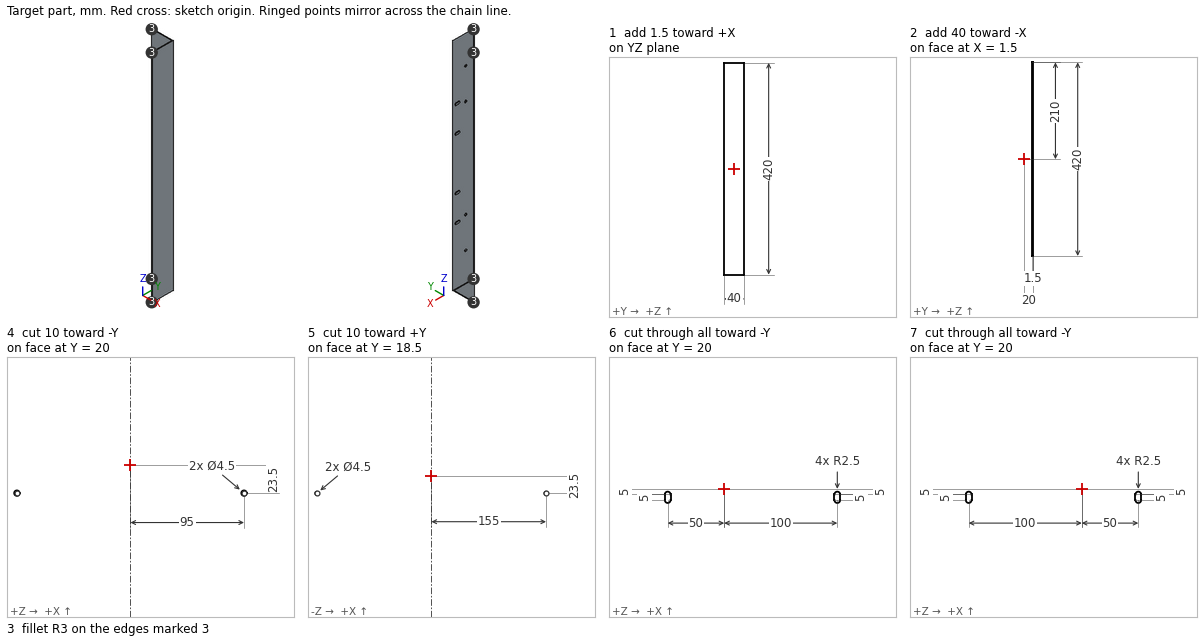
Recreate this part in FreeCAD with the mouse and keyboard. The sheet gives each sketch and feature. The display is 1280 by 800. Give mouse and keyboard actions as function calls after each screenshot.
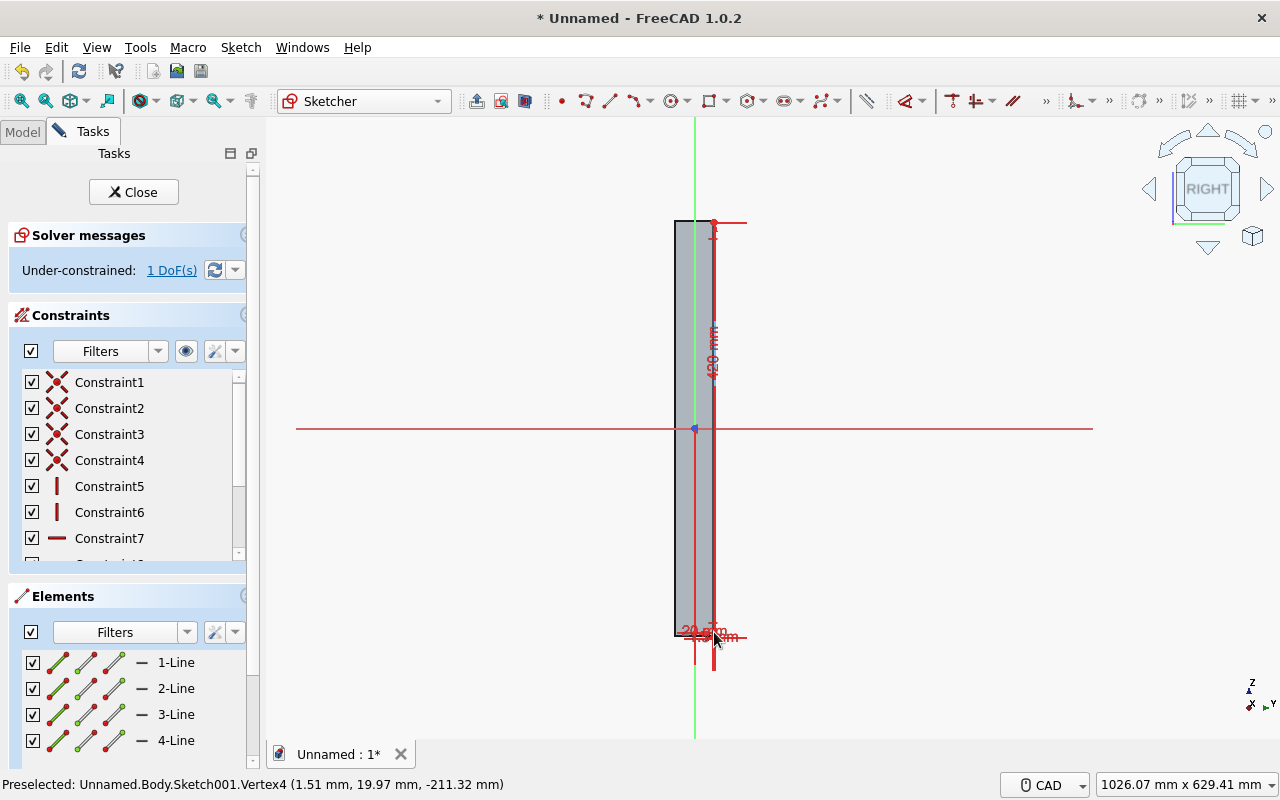
scroll(713, 223, up, 11)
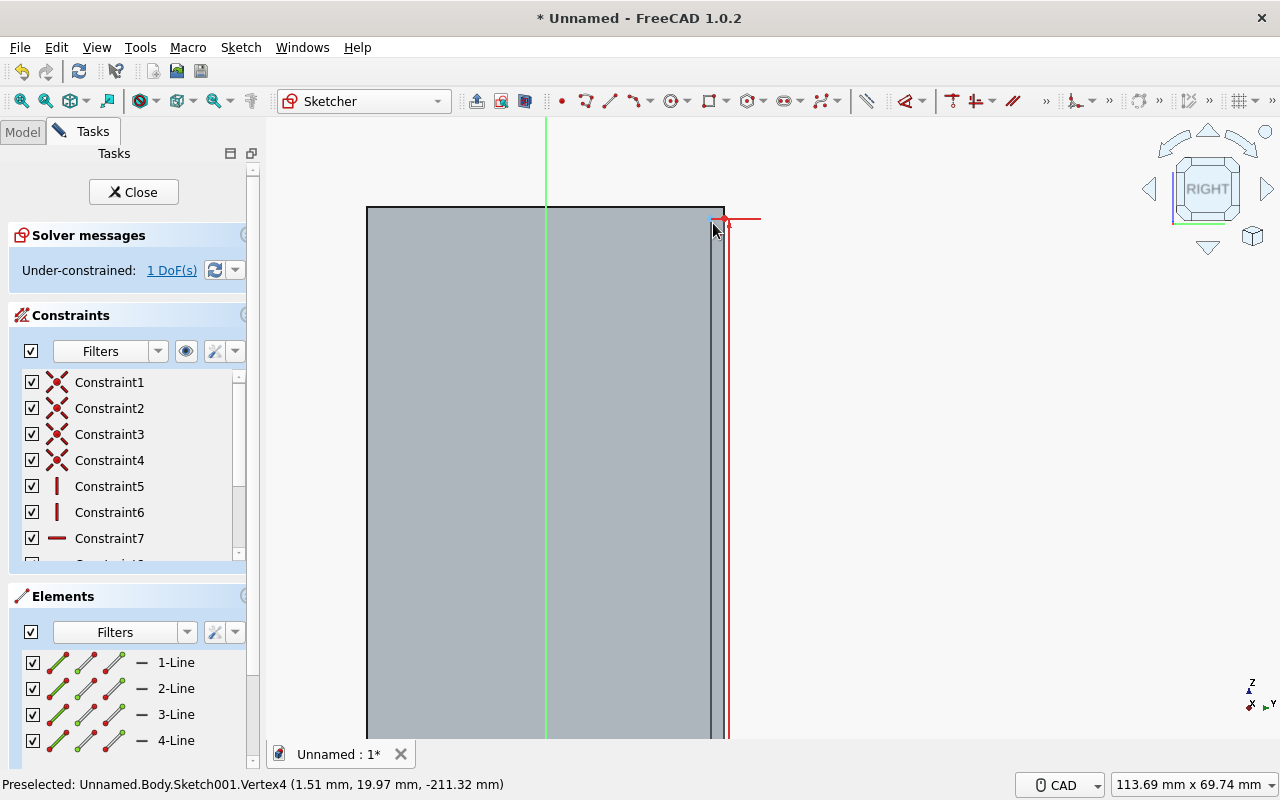
click(711, 219)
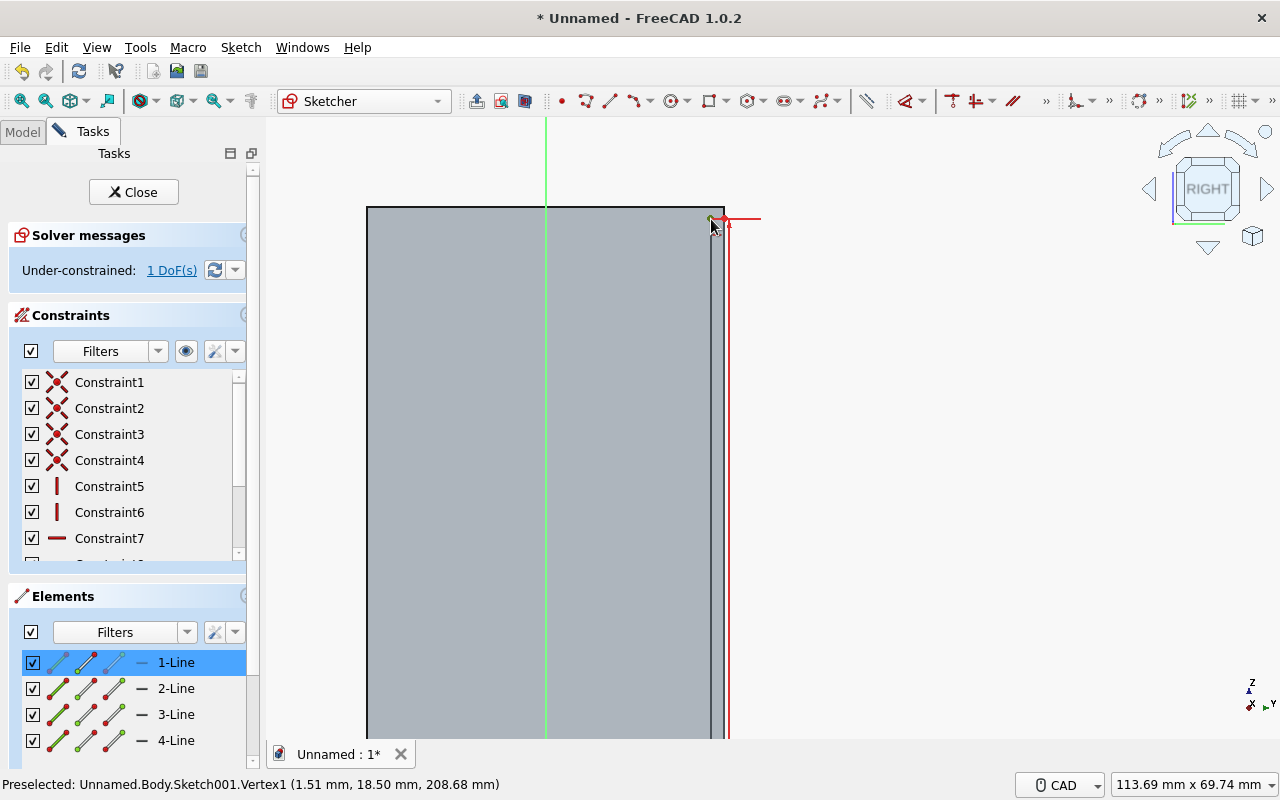
key(i)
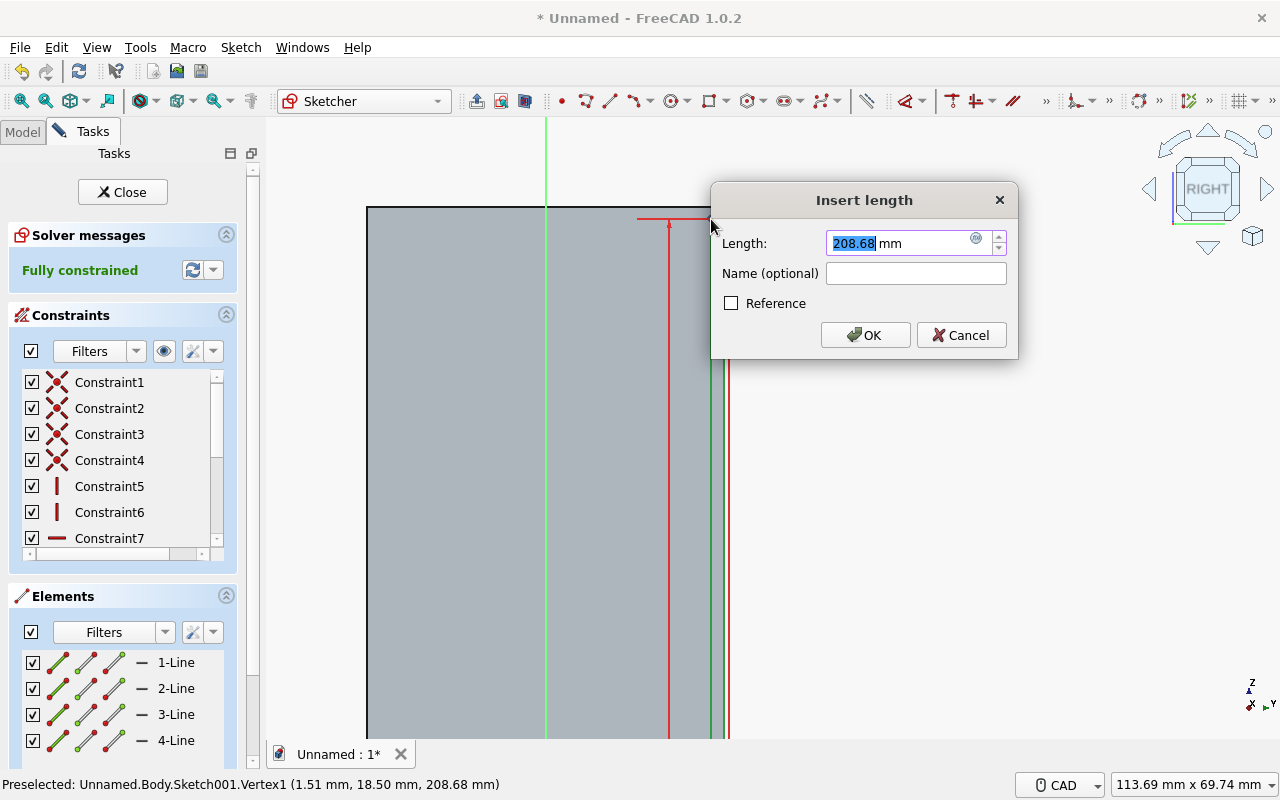
text(210)
key(Return)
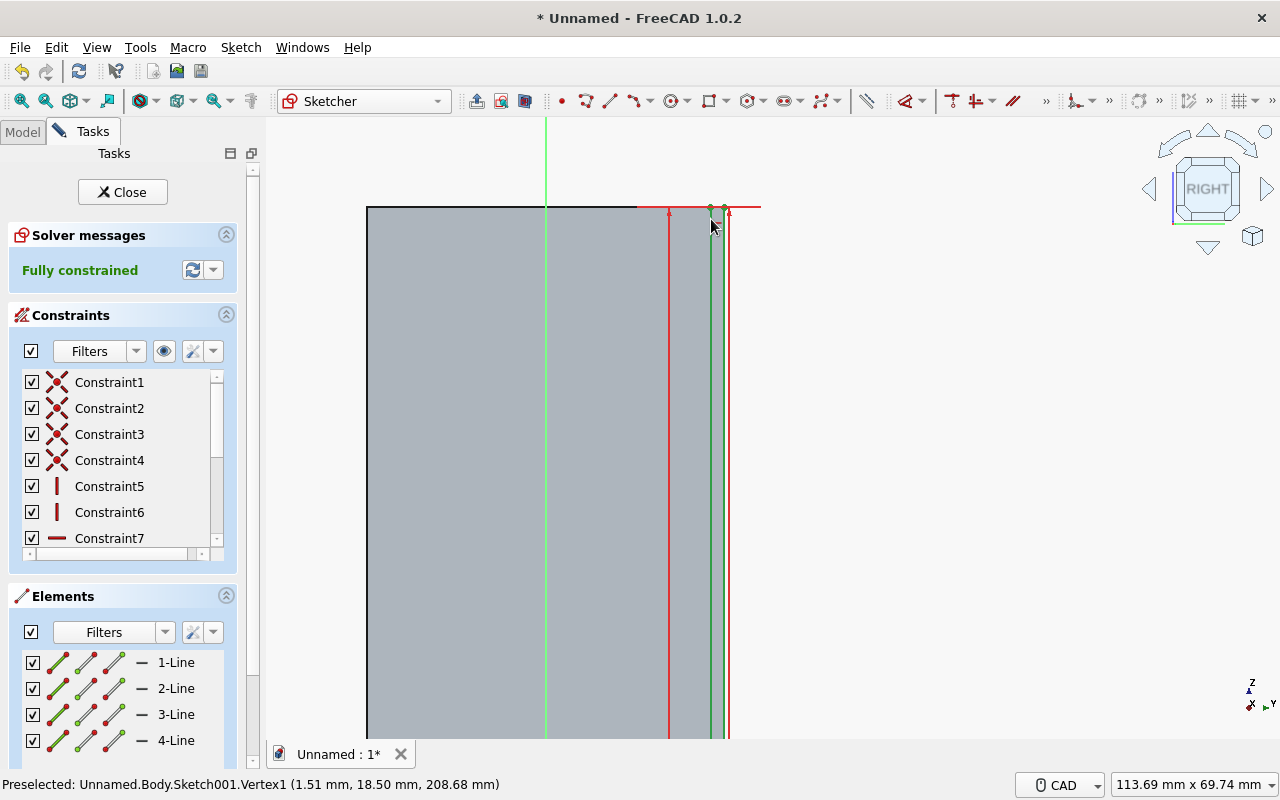
click(123, 192)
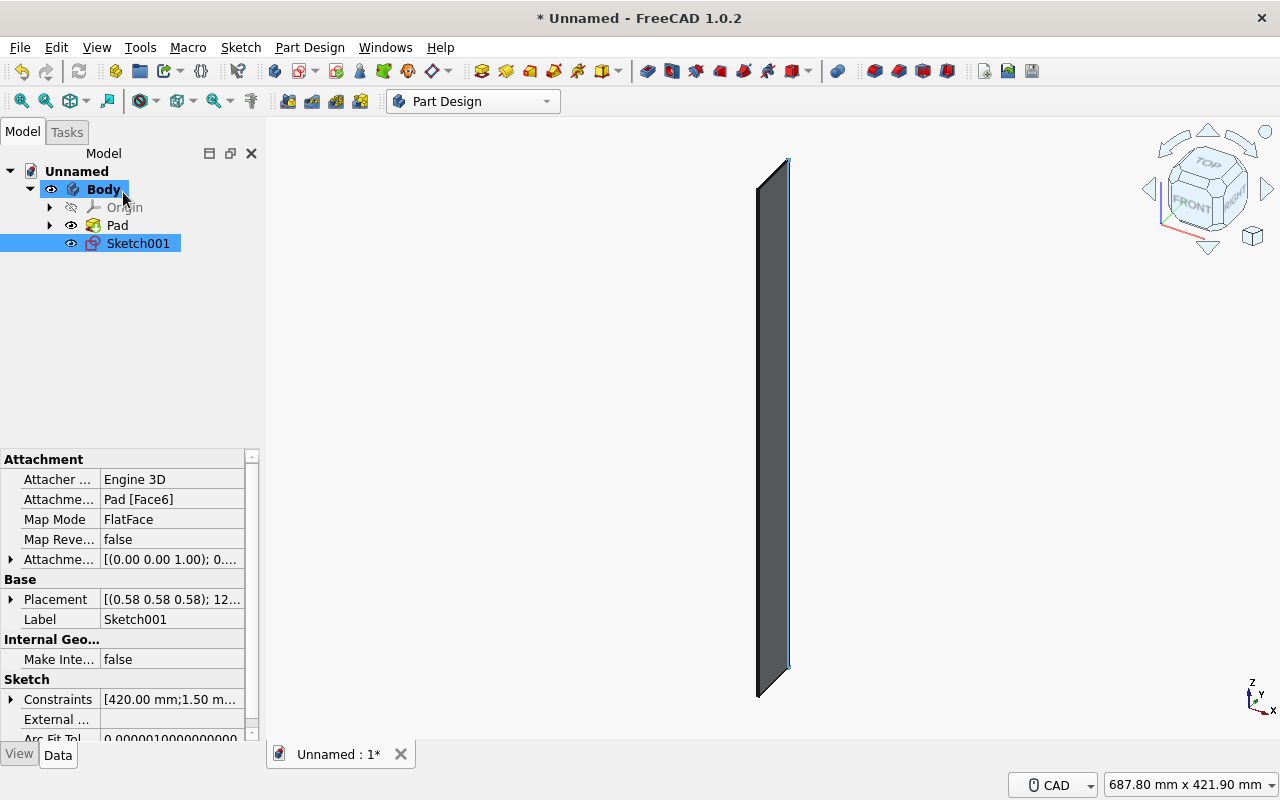
click(482, 72)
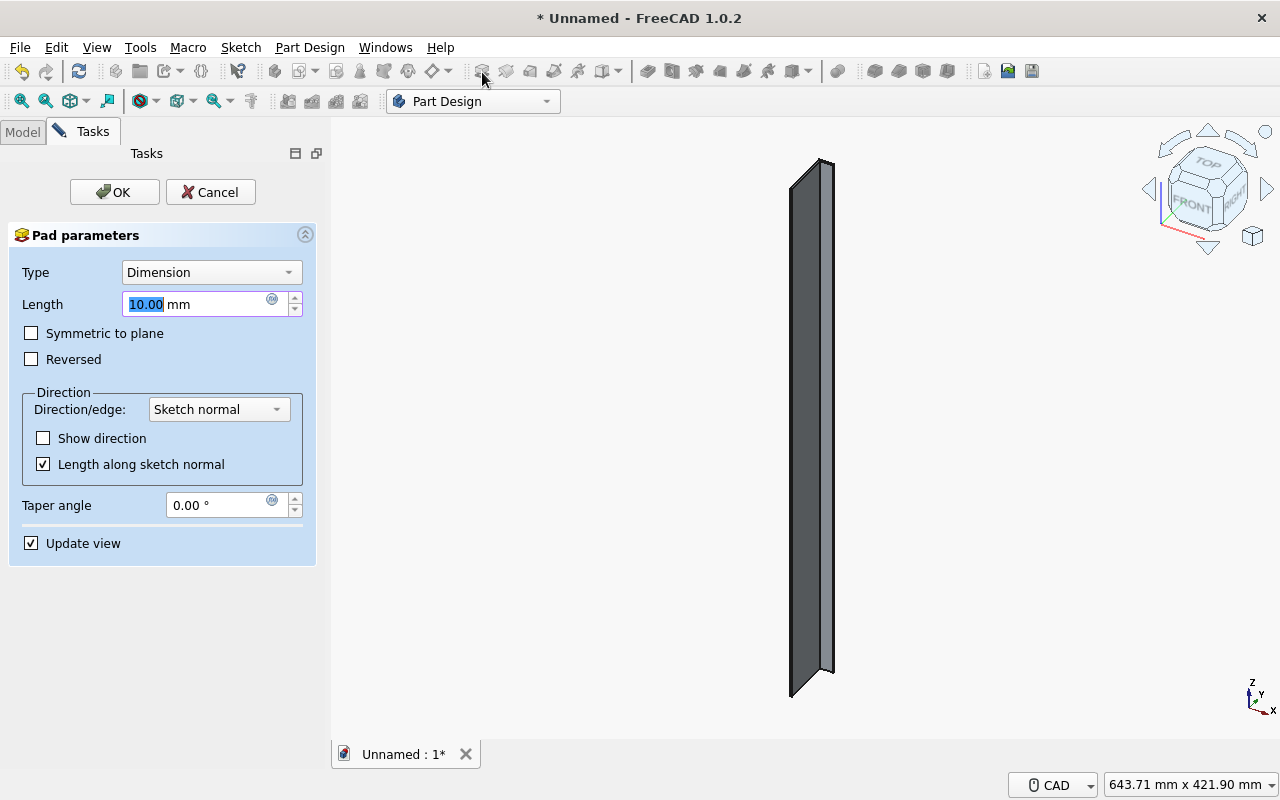
text(40)
key(Tab)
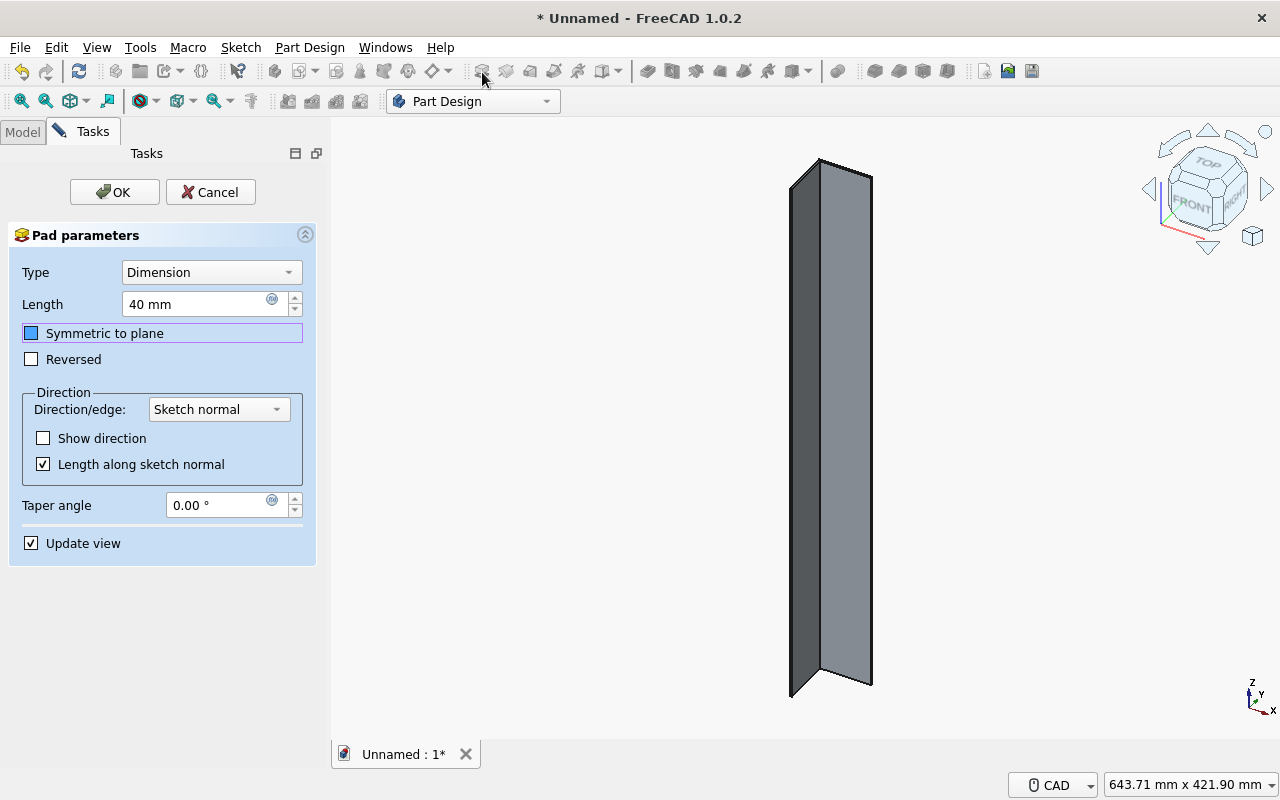
click(30, 359)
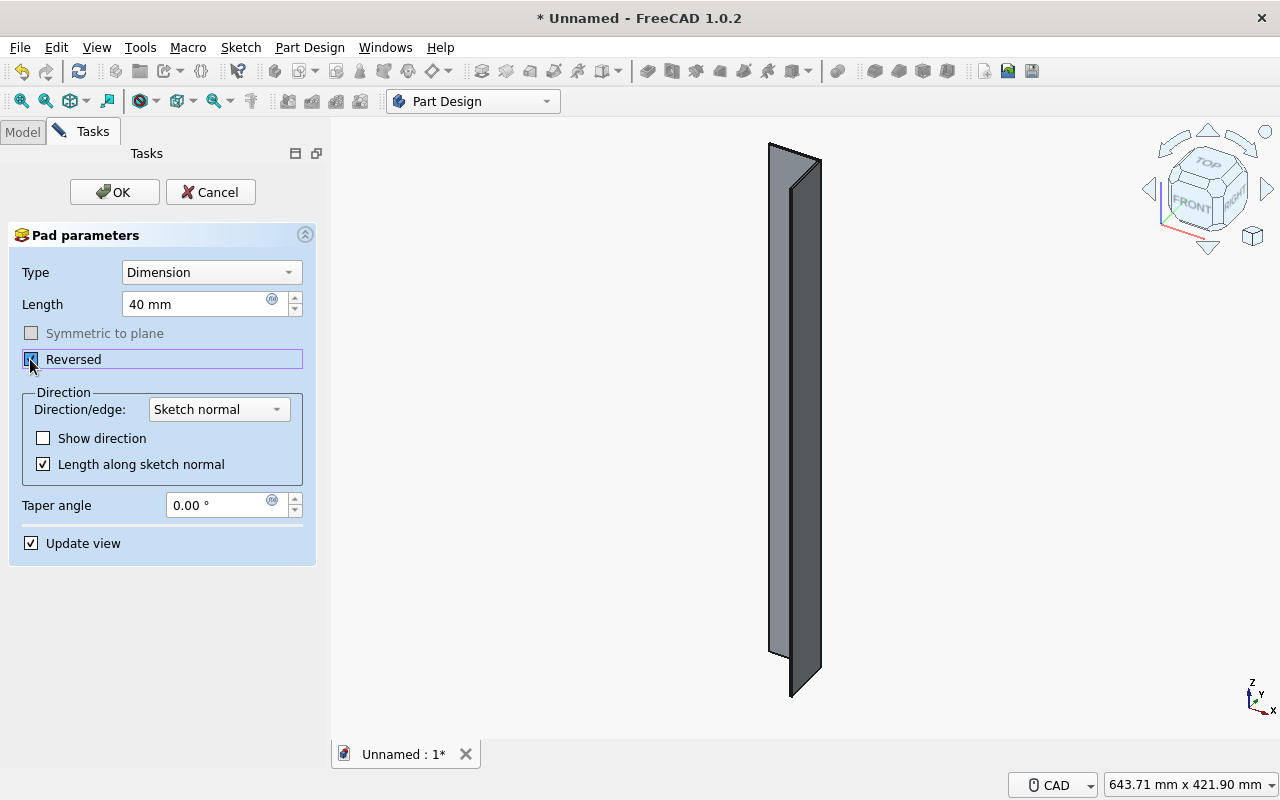
click(115, 192)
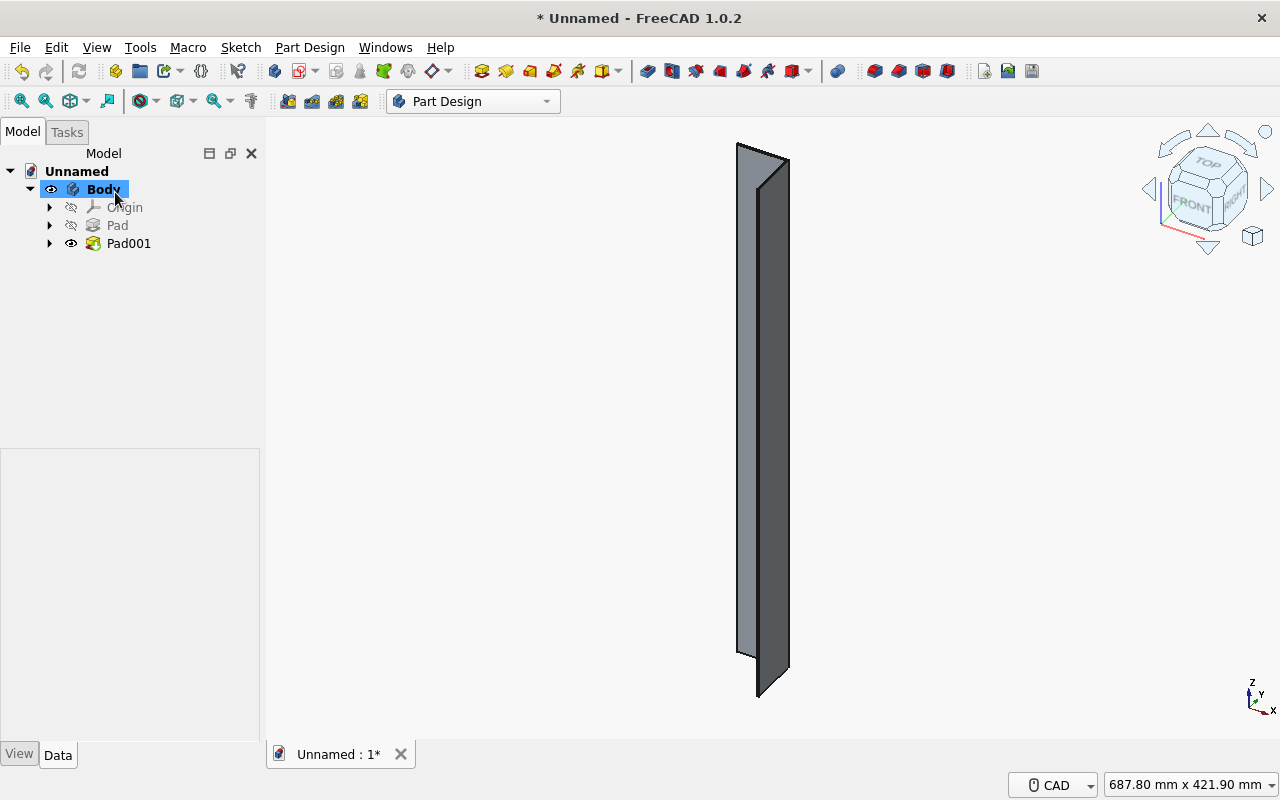
key(0)